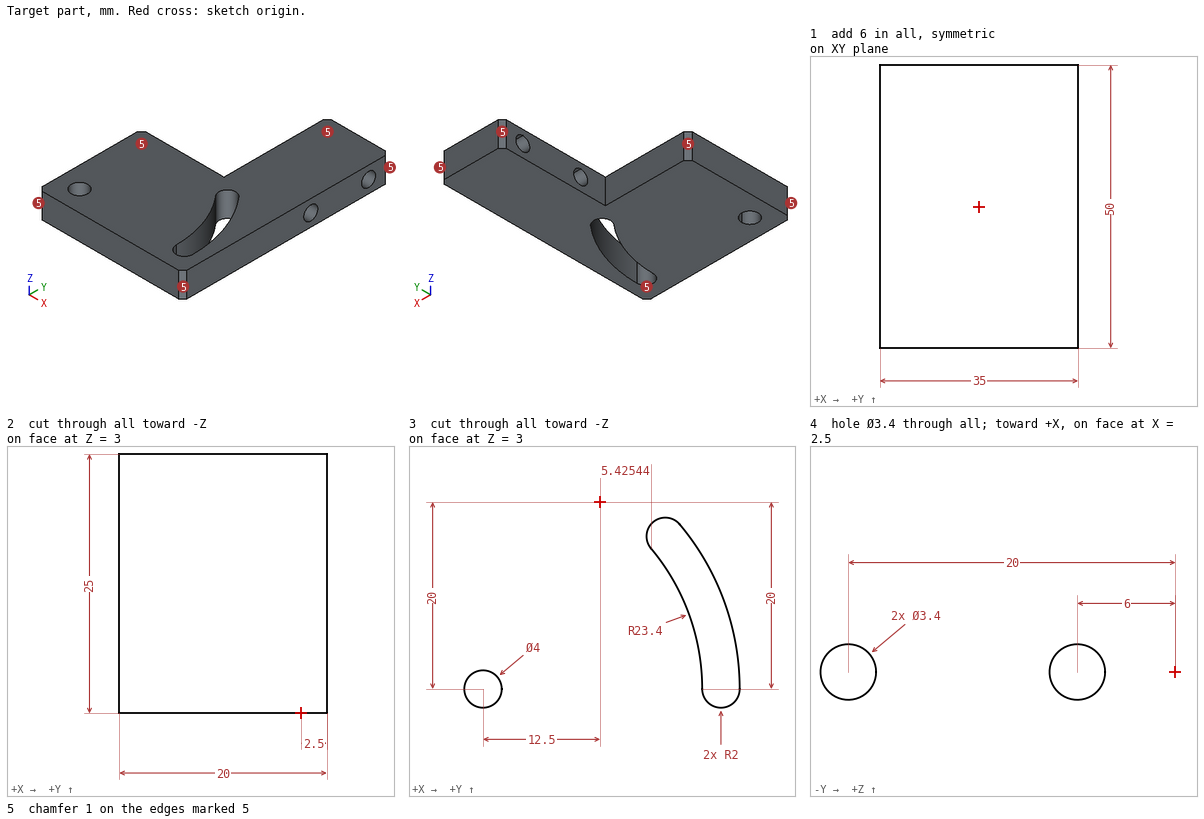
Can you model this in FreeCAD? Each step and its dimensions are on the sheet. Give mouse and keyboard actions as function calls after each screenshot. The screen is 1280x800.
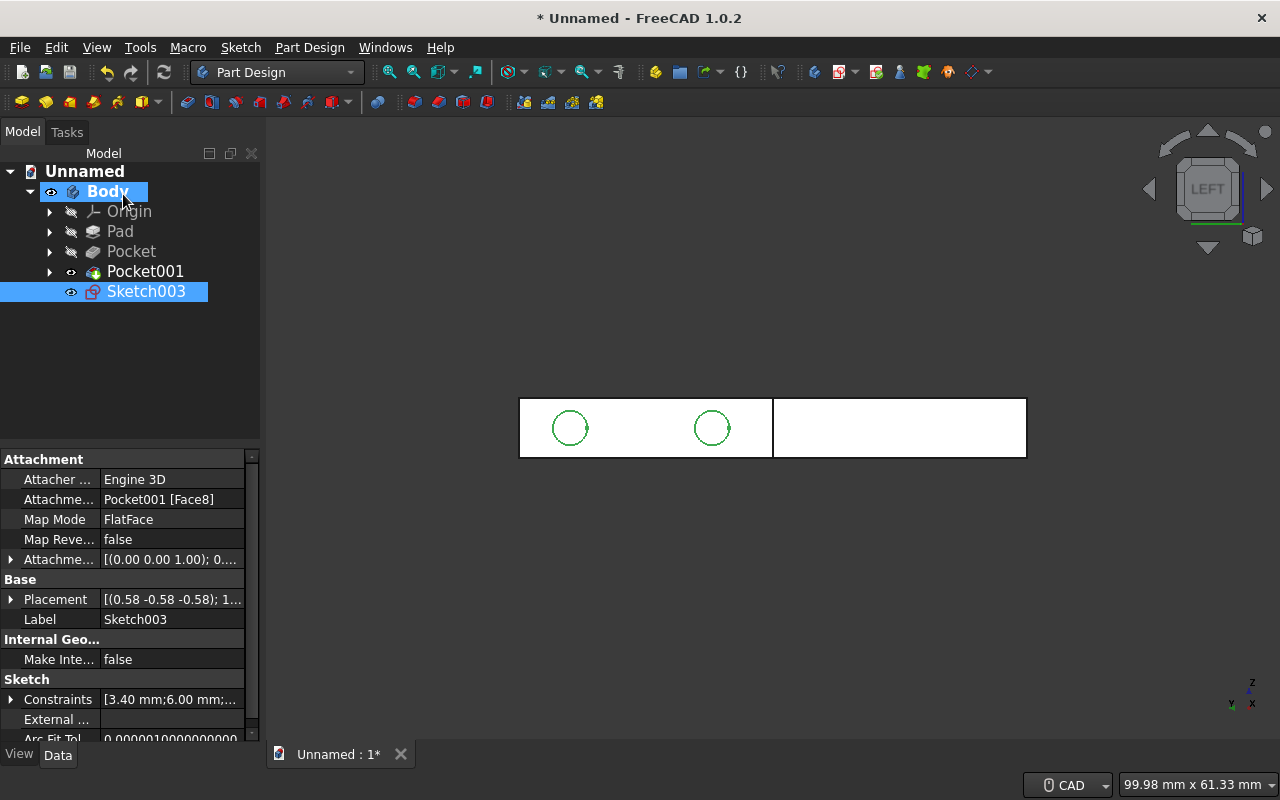
click(212, 102)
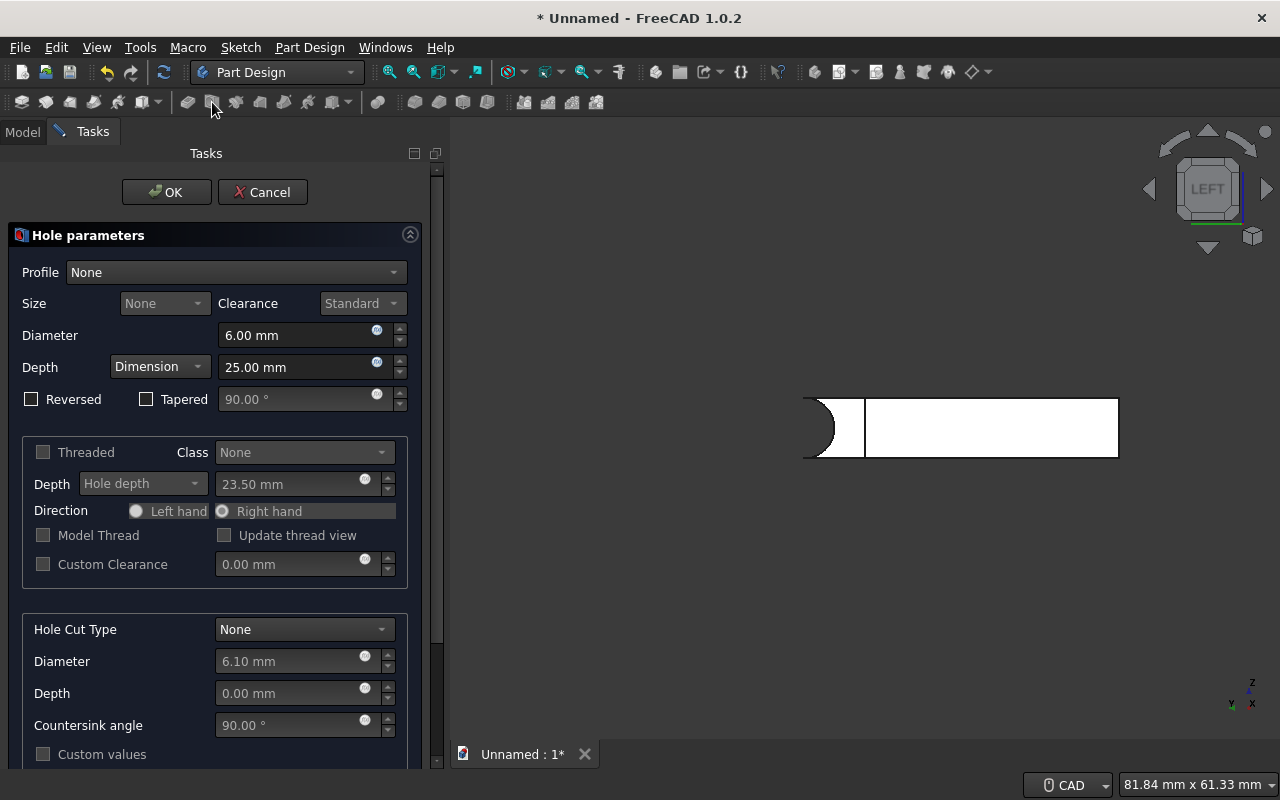
triple_click(305, 335)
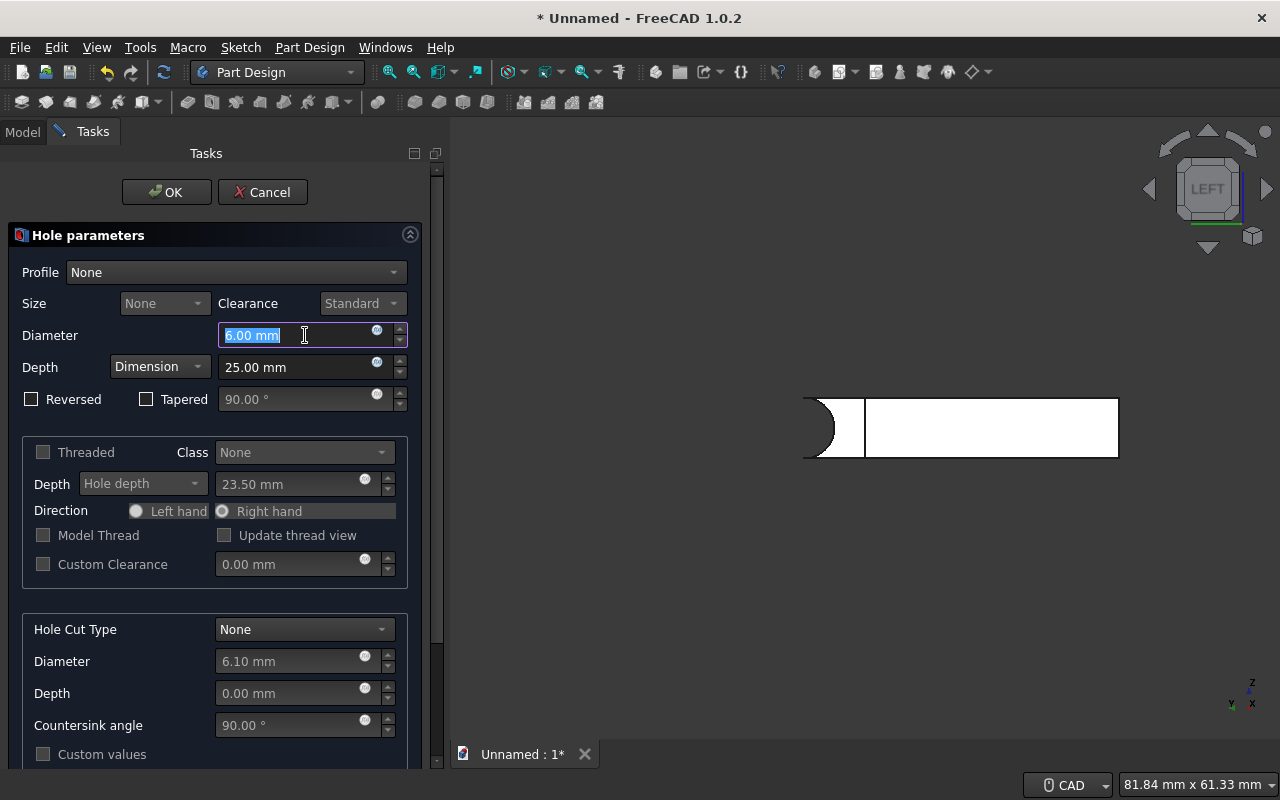
text(3.4)
key(Tab)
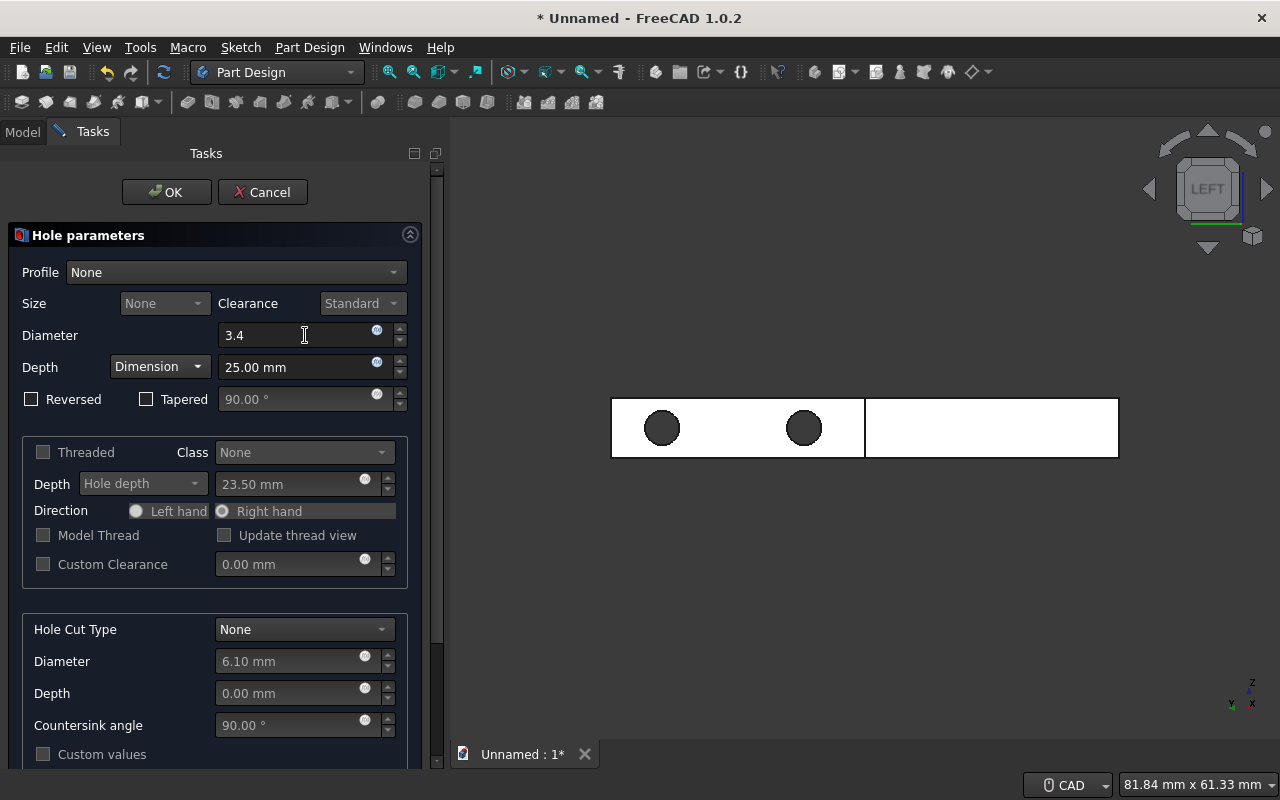
click(161, 366)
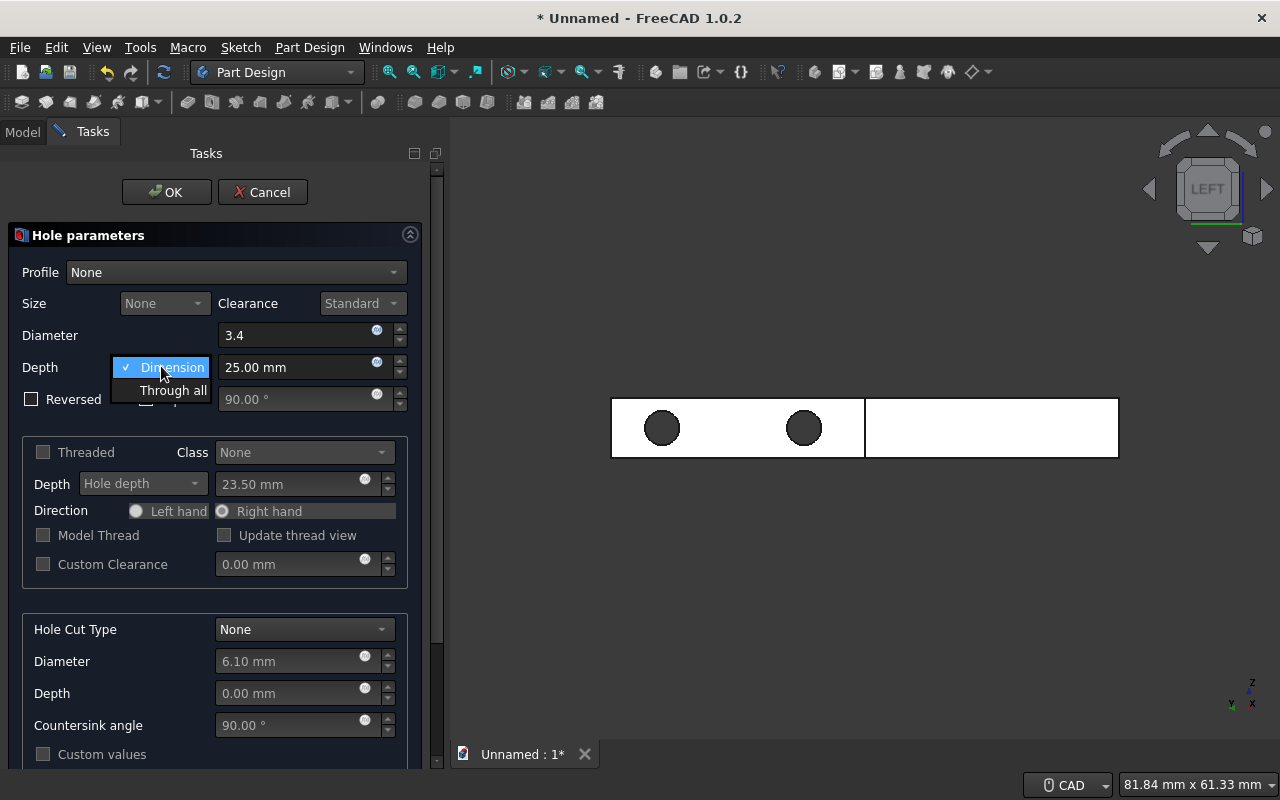
click(160, 390)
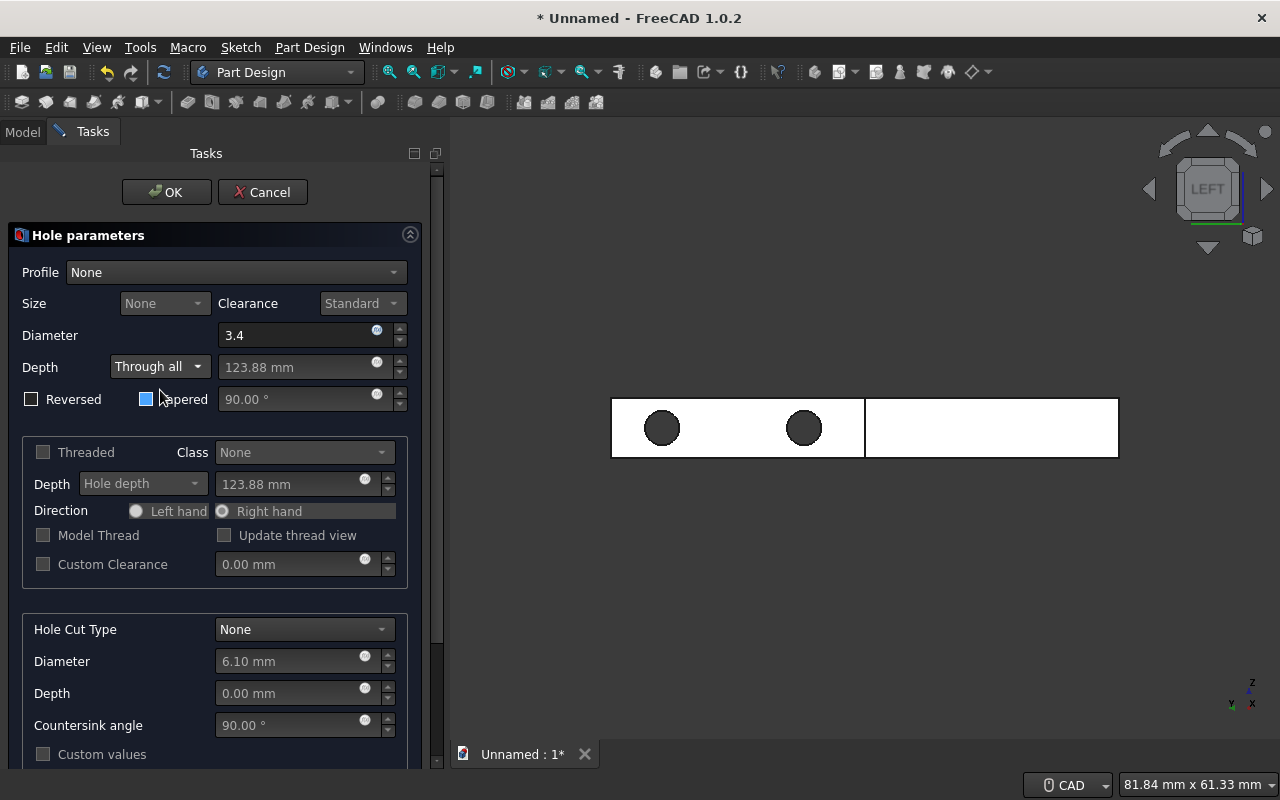
click(167, 192)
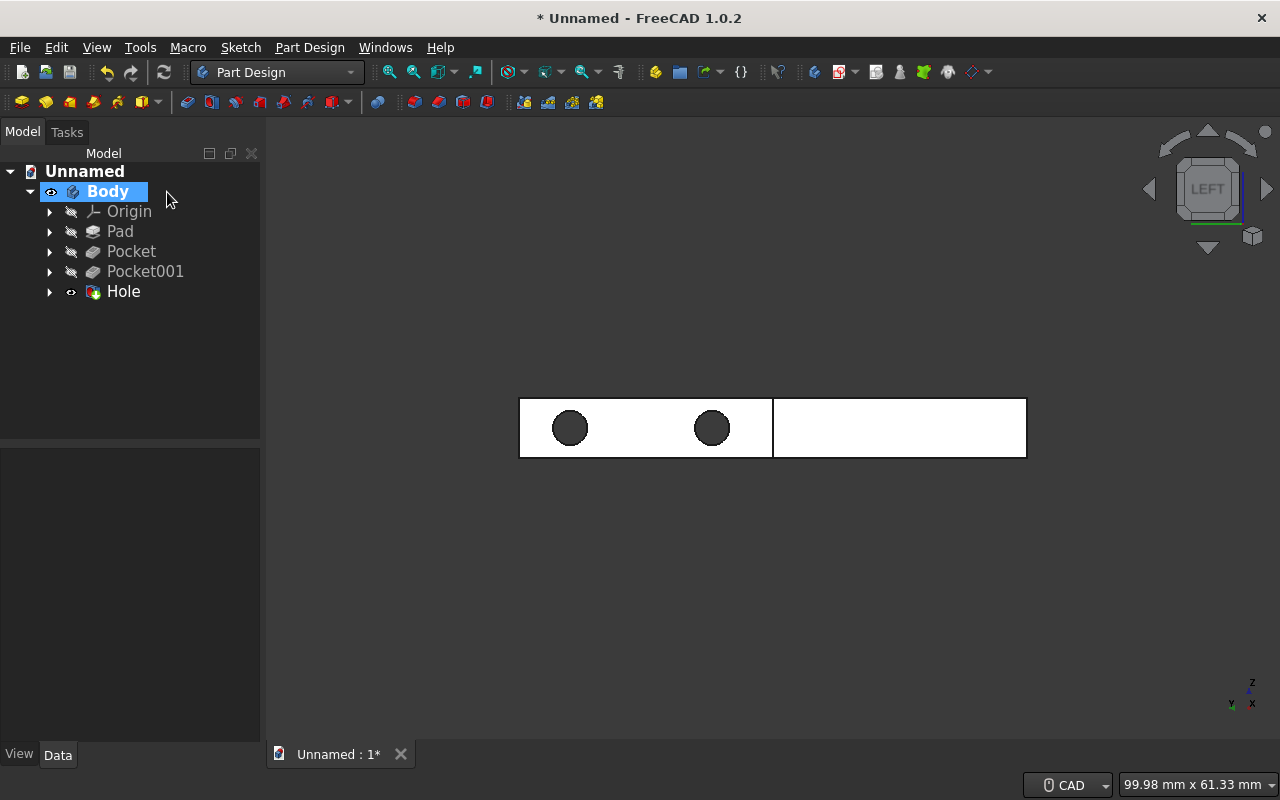
click(773, 427)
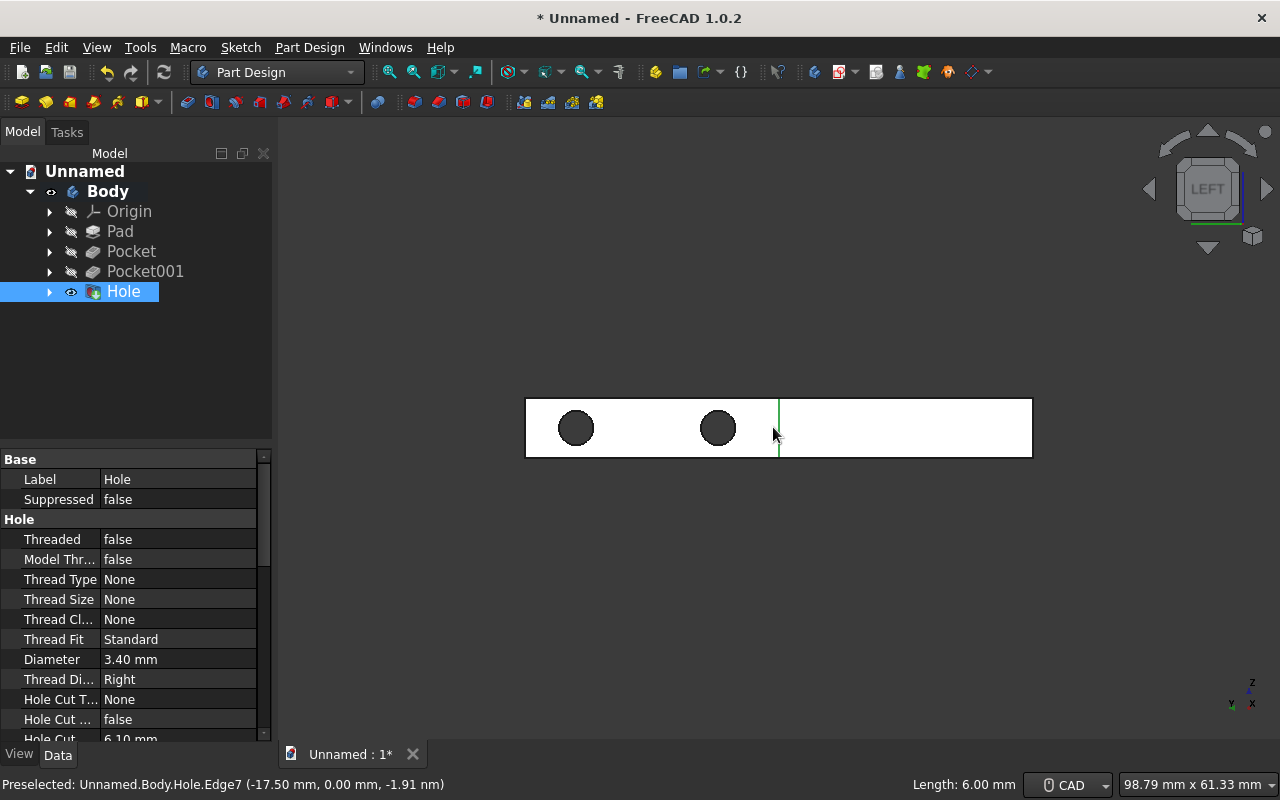
click(525, 427, ctrl)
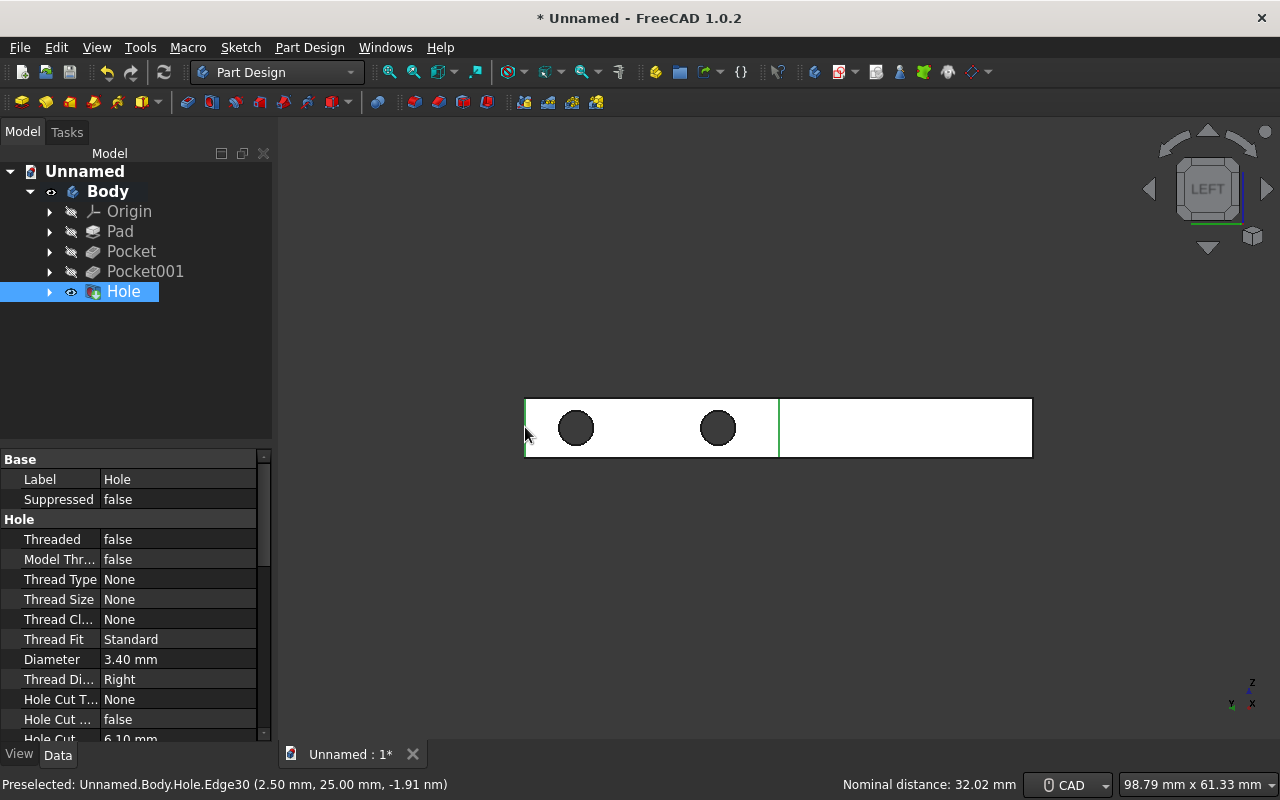
click(1033, 427, ctrl)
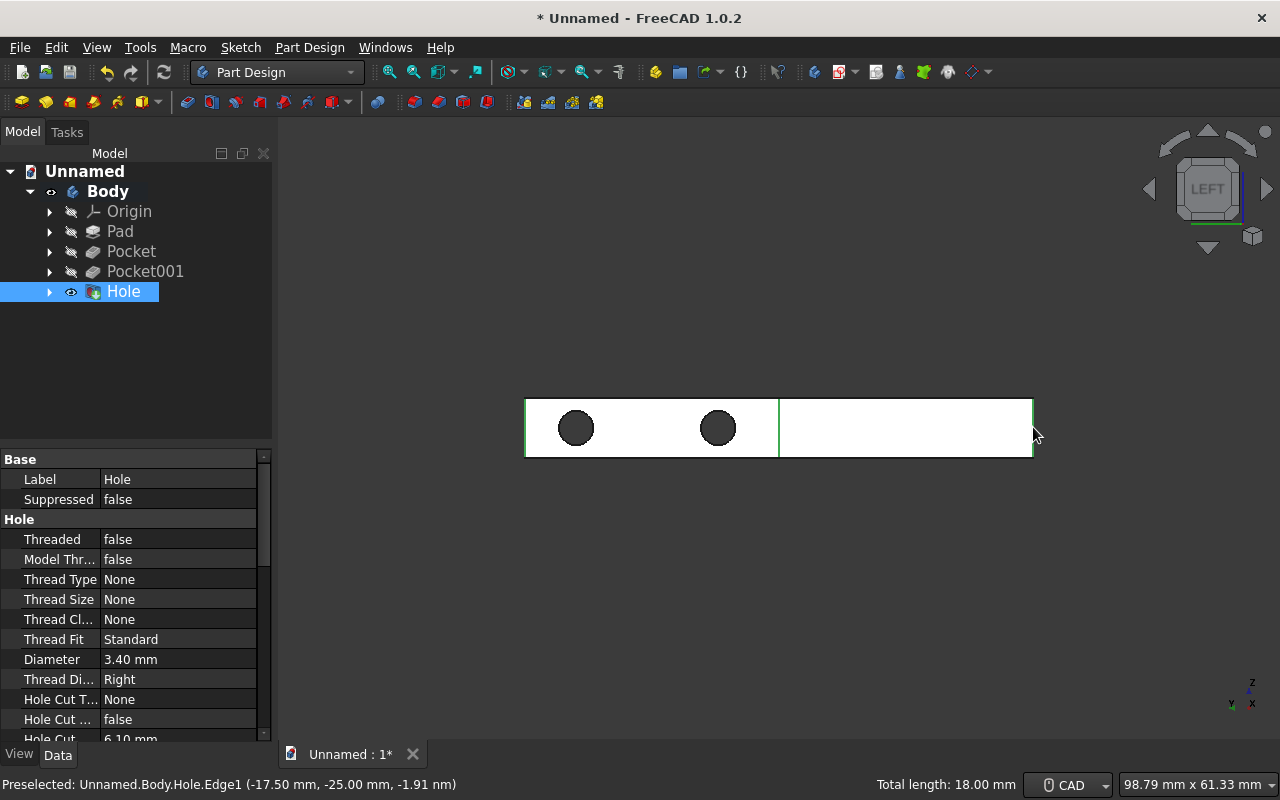
key(0)